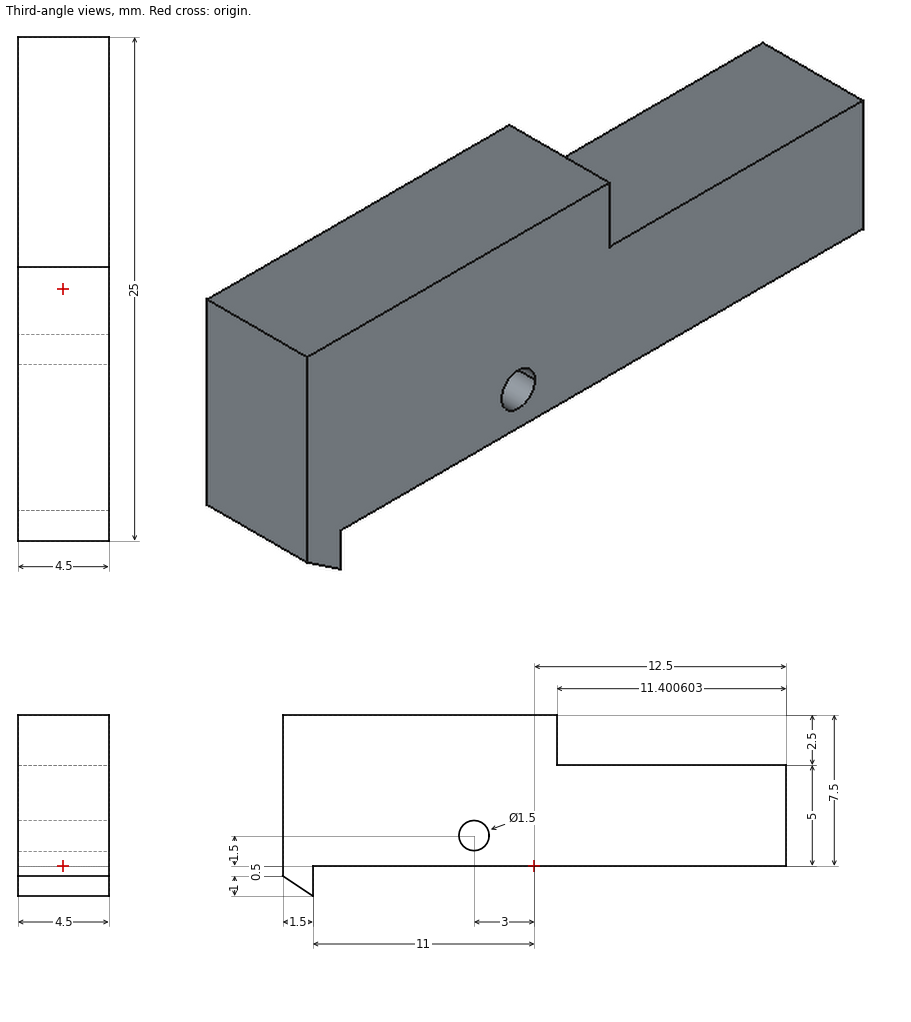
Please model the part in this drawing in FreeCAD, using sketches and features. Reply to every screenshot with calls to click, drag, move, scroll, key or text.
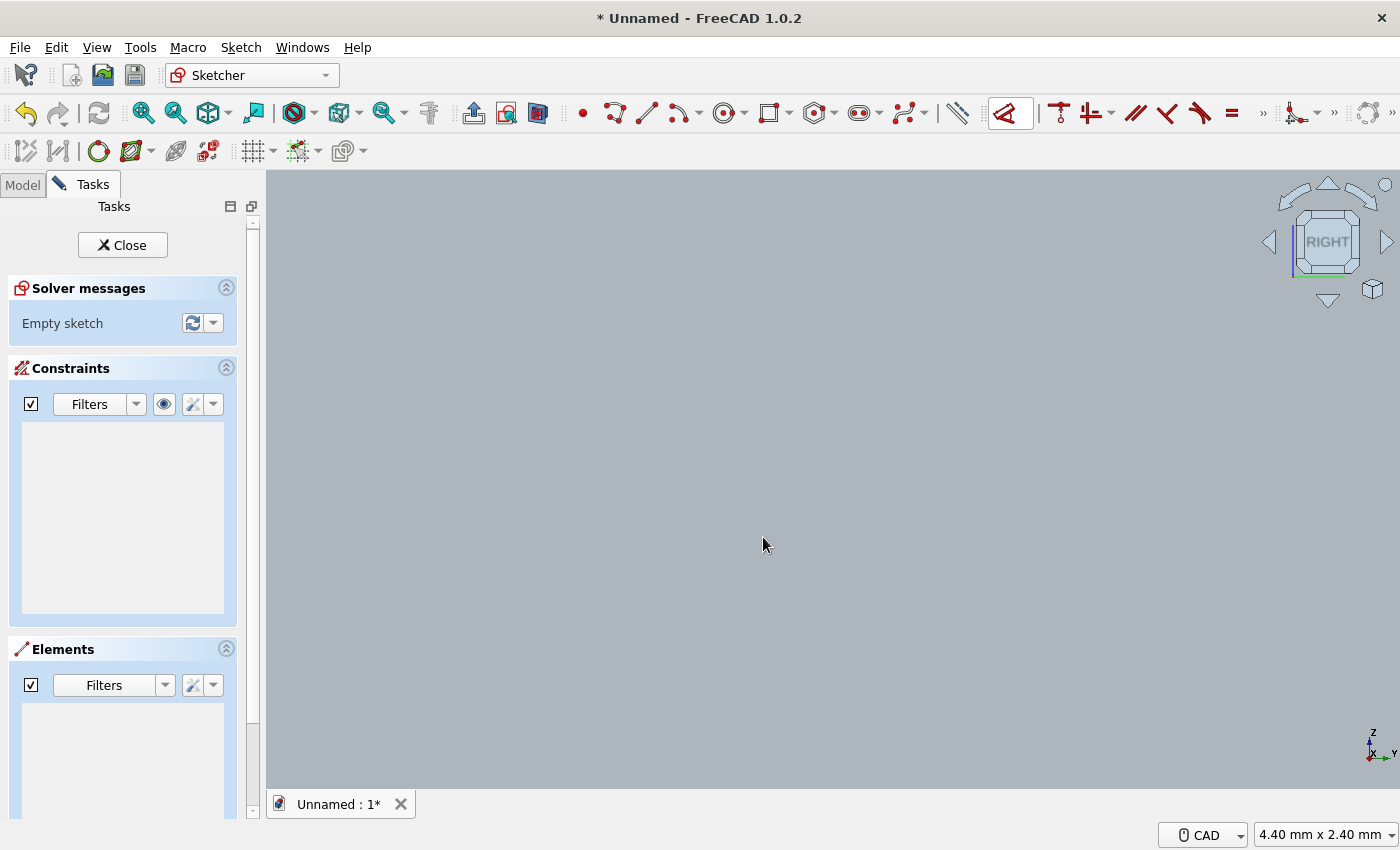
click(724, 114)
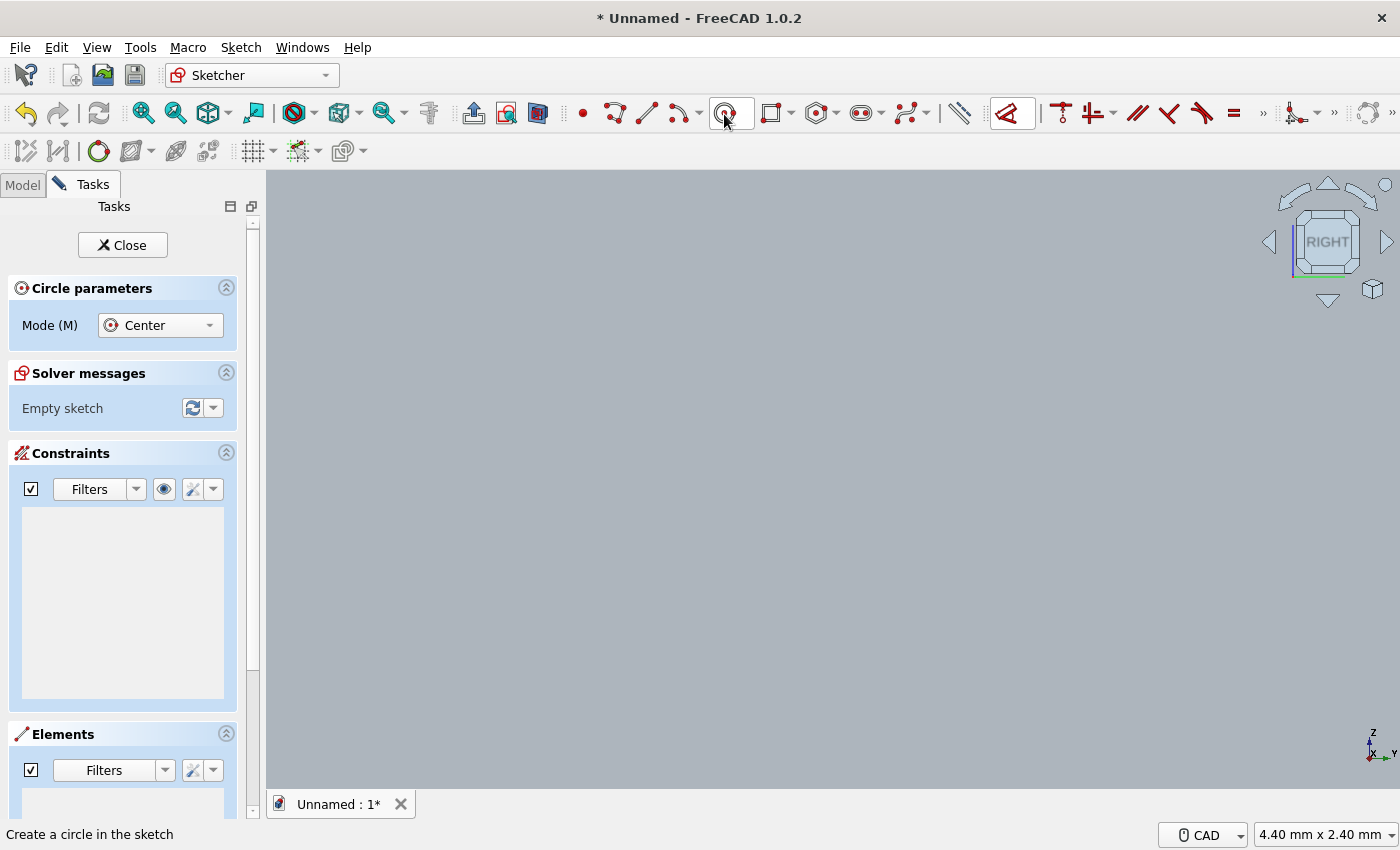
click(757, 477)
move(894, 340)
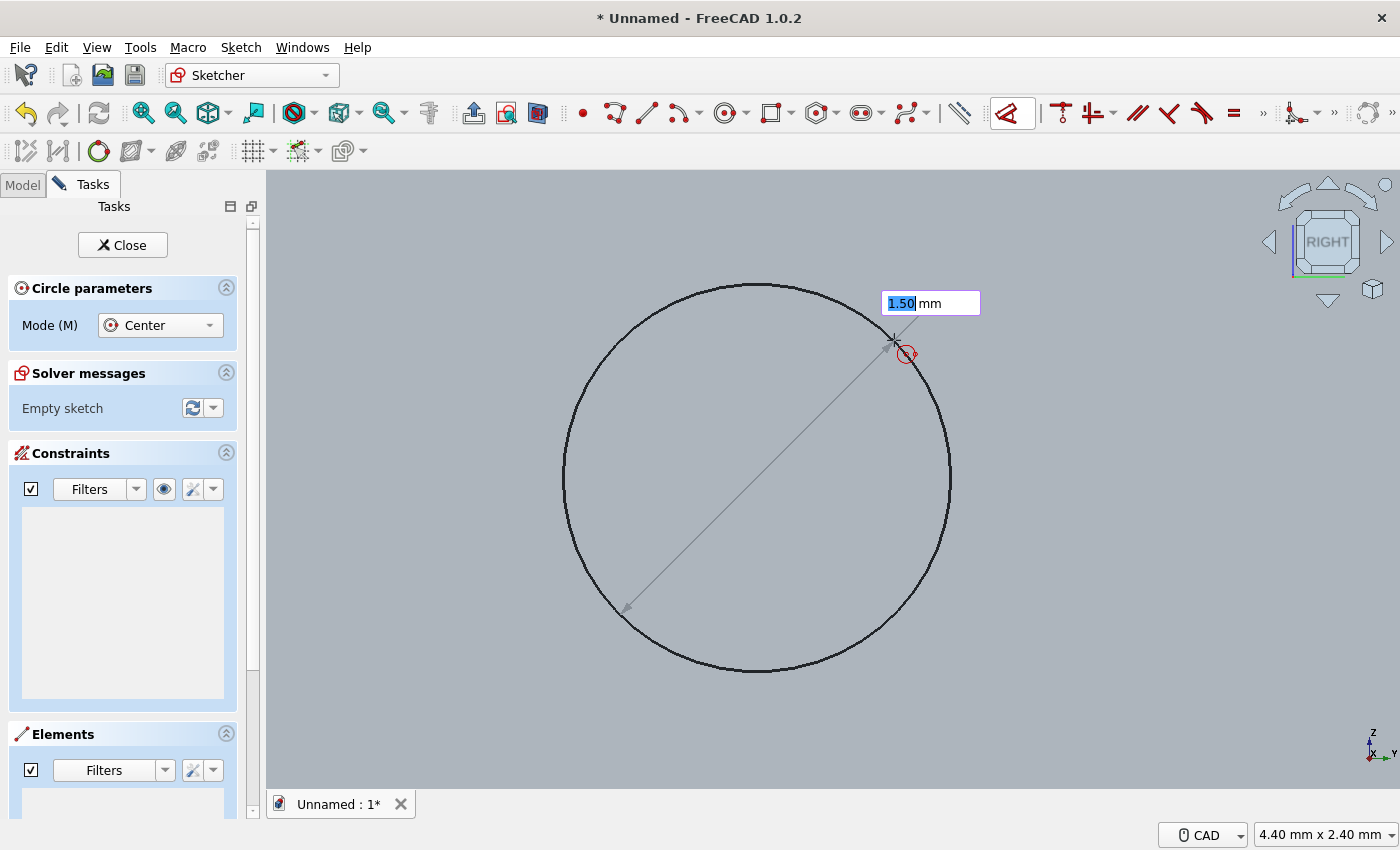
text(1.5)
key(Return)
key(Escape)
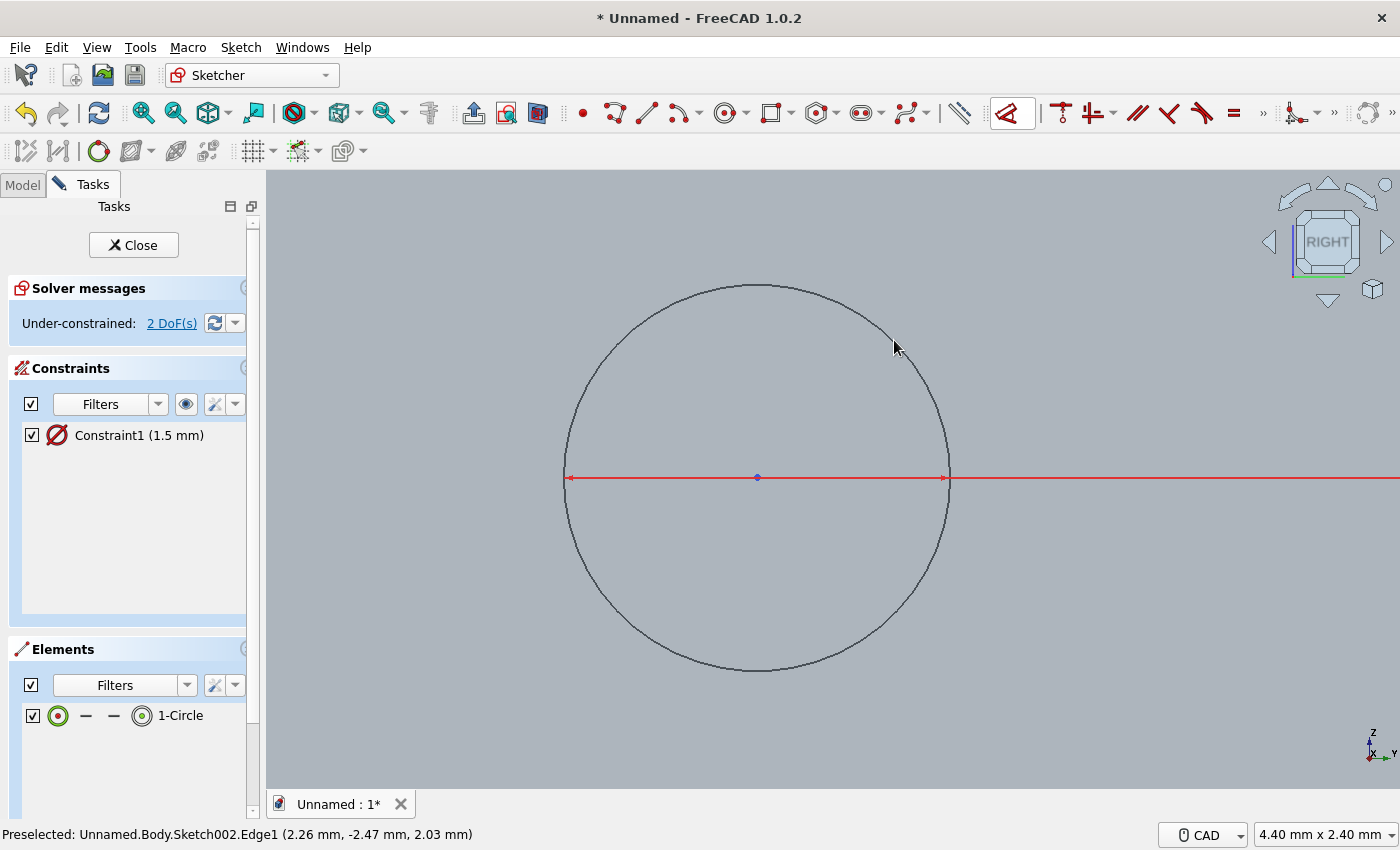
click(757, 478)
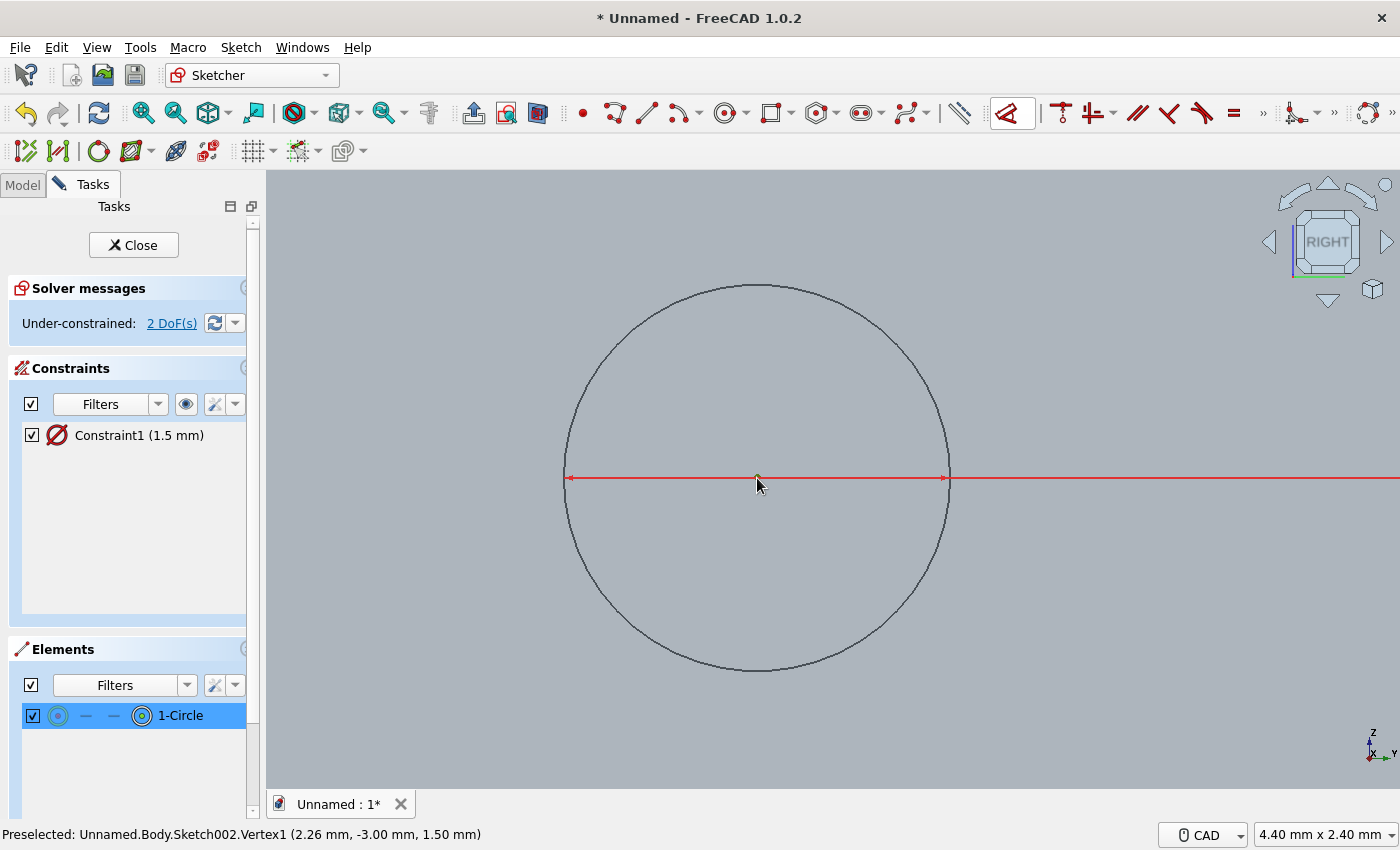
key(l)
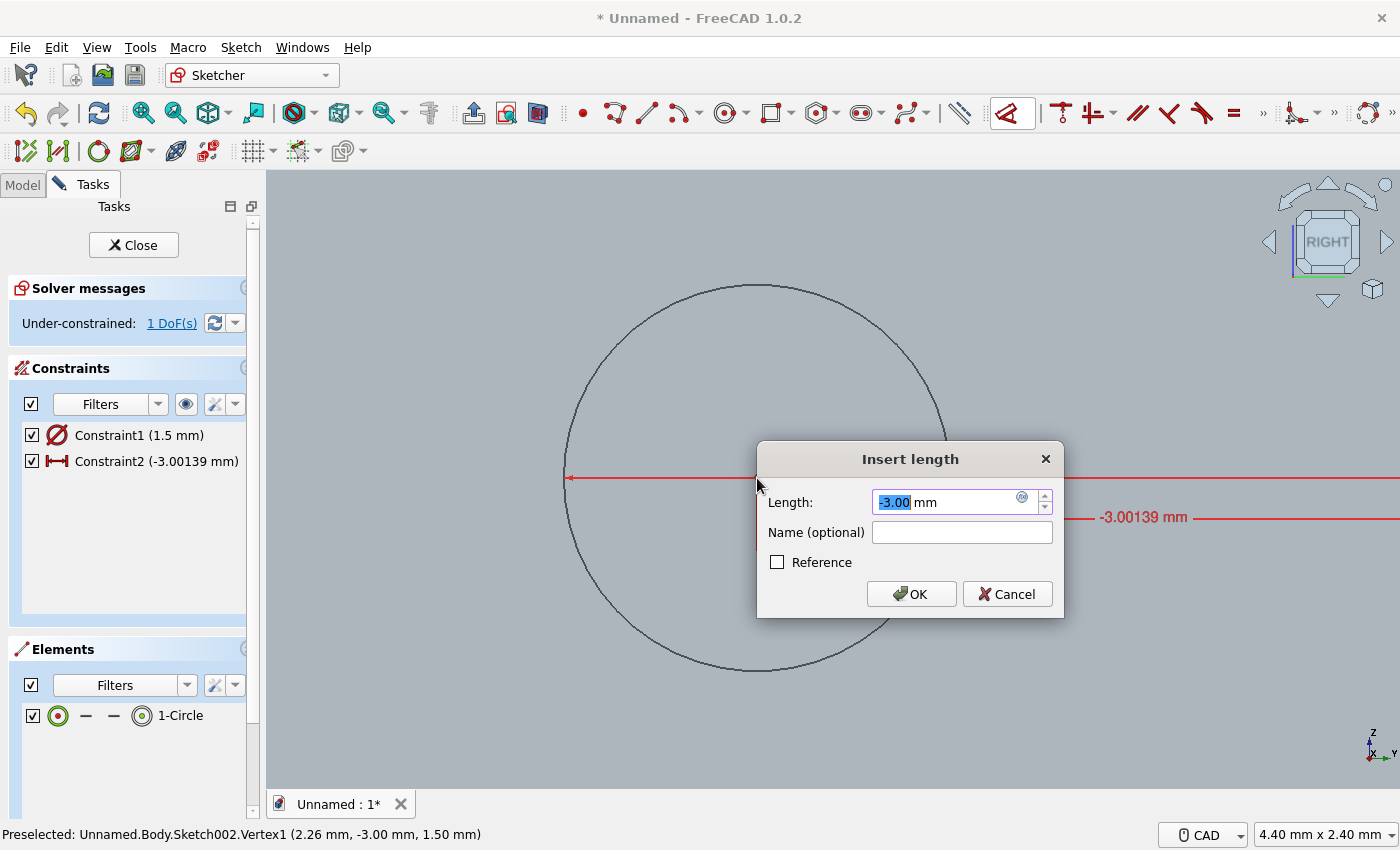
text(-3)
key(Return)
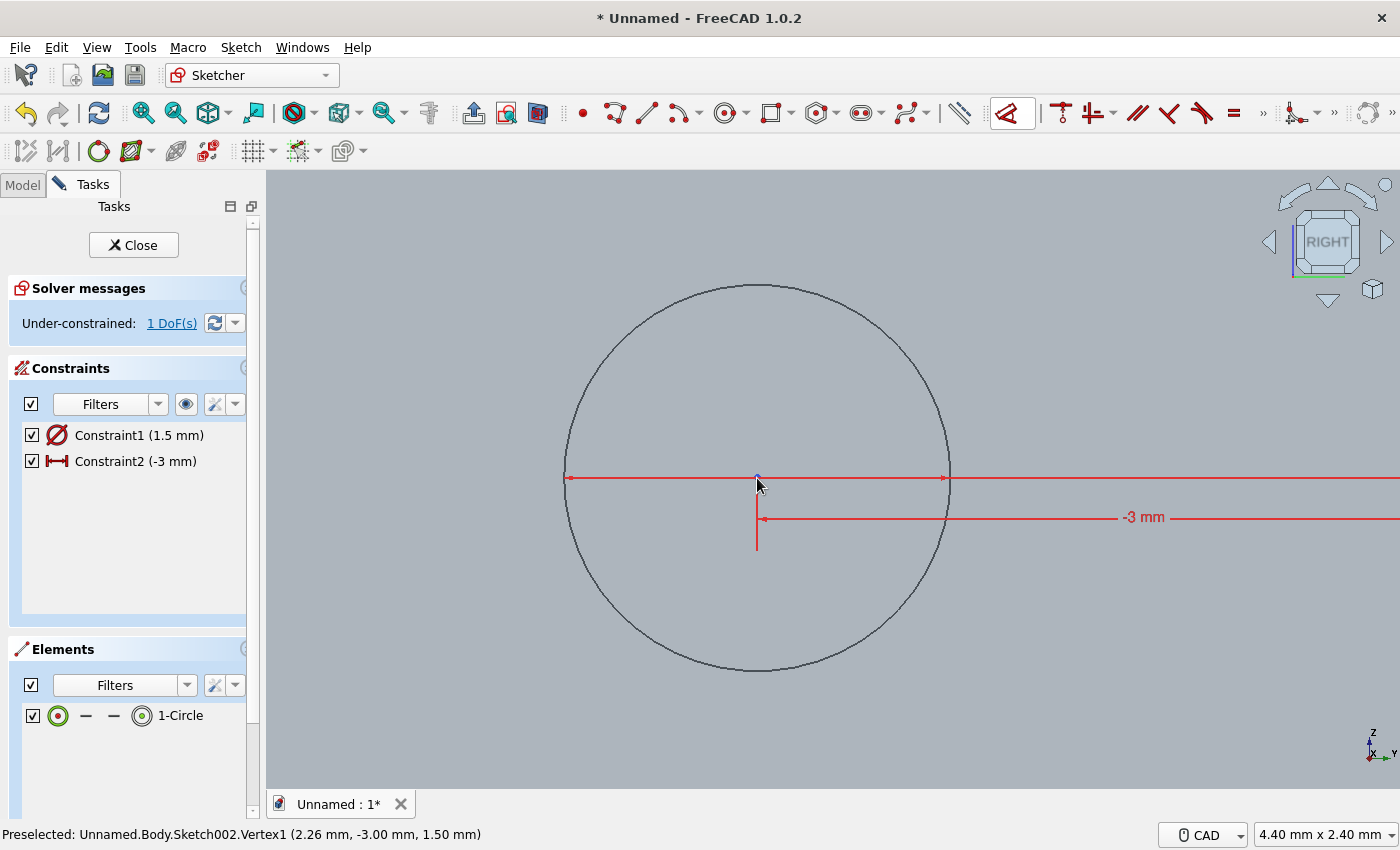
click(757, 478)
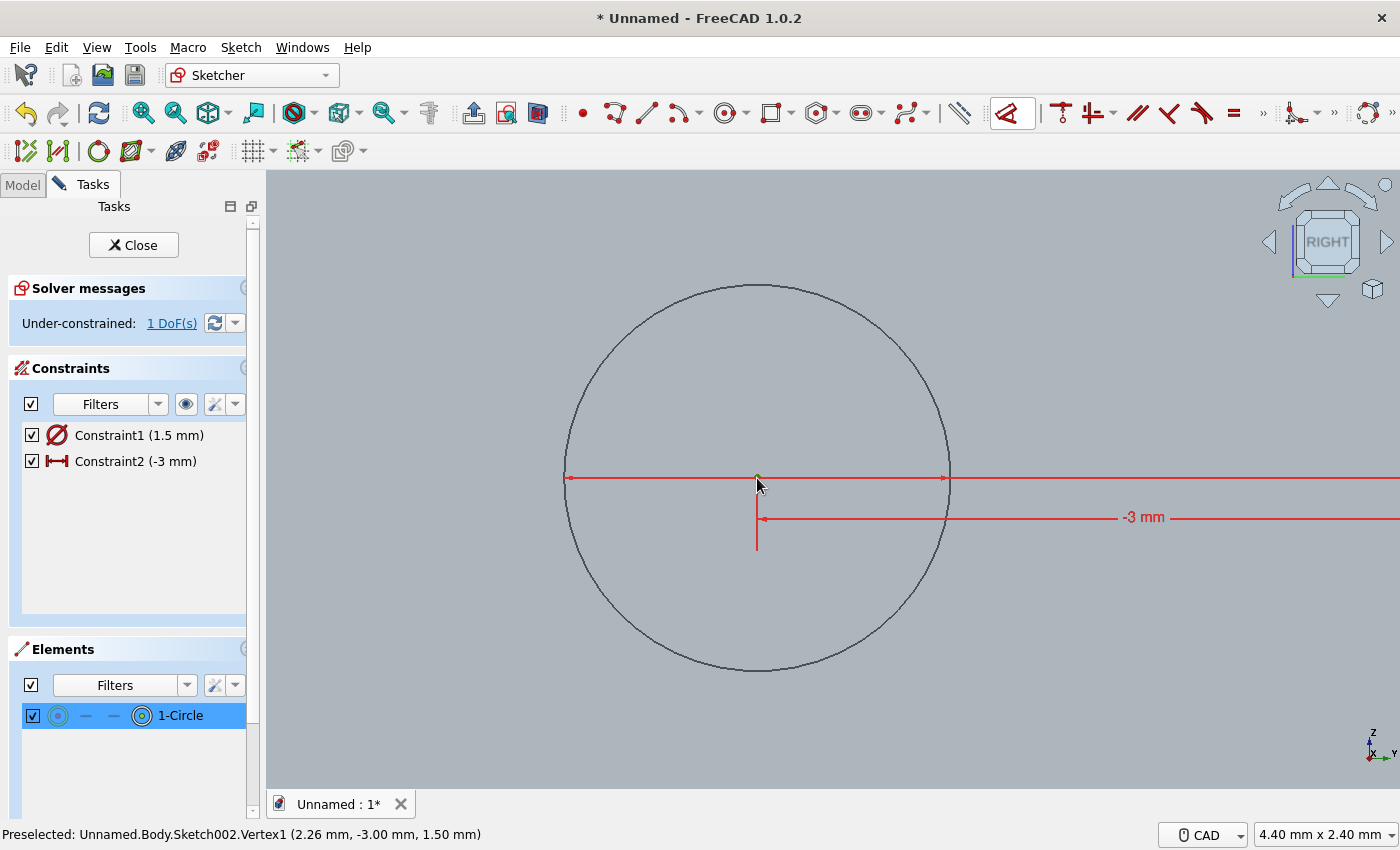
key(i)